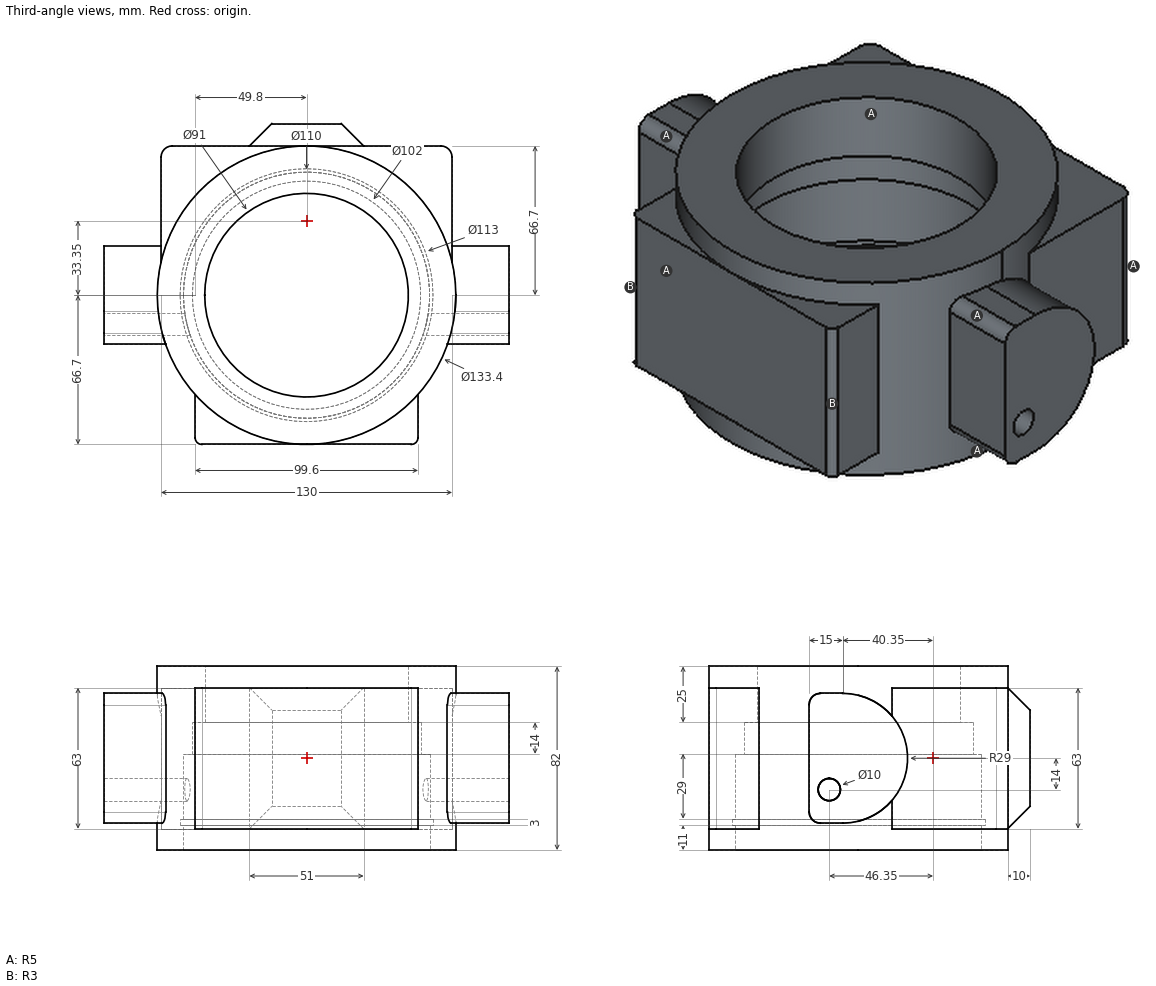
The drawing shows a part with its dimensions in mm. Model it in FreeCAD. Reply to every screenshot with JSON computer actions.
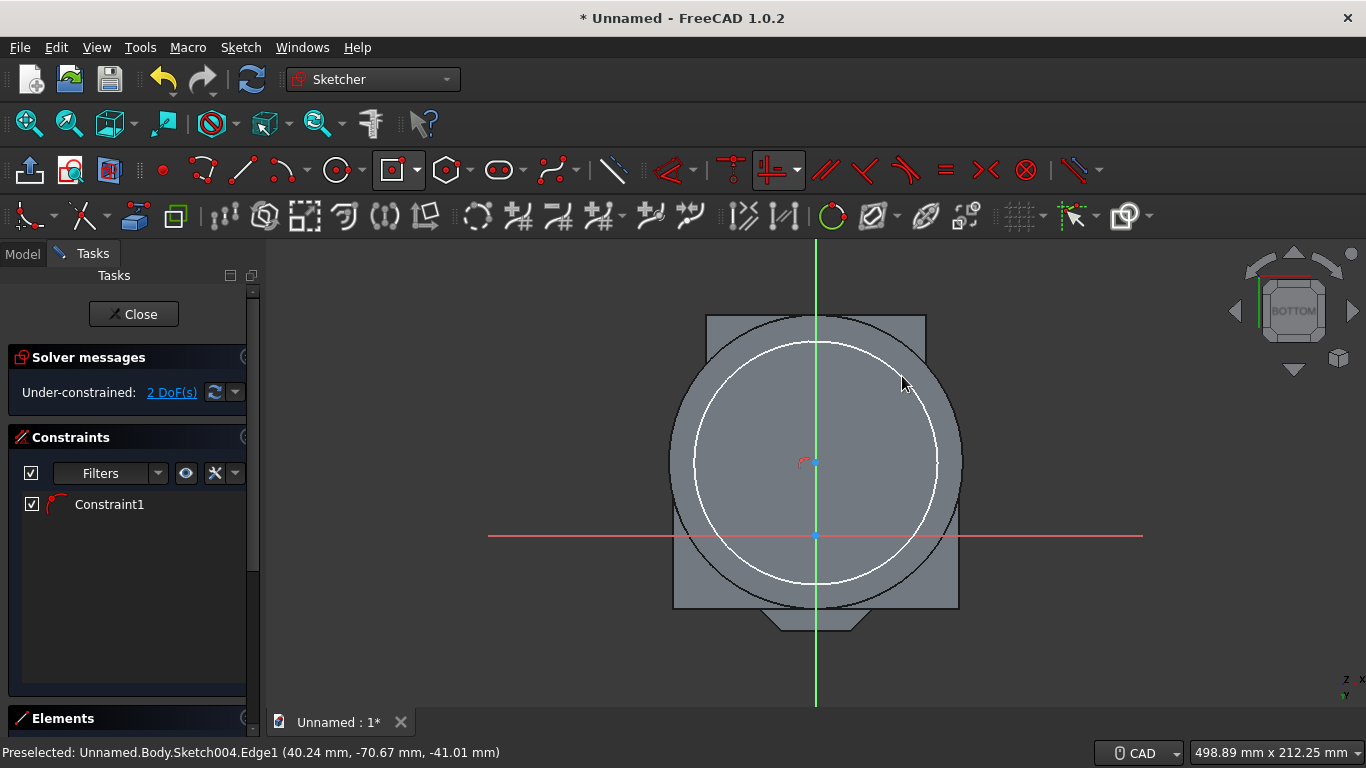
{"action": "key", "text": "d"}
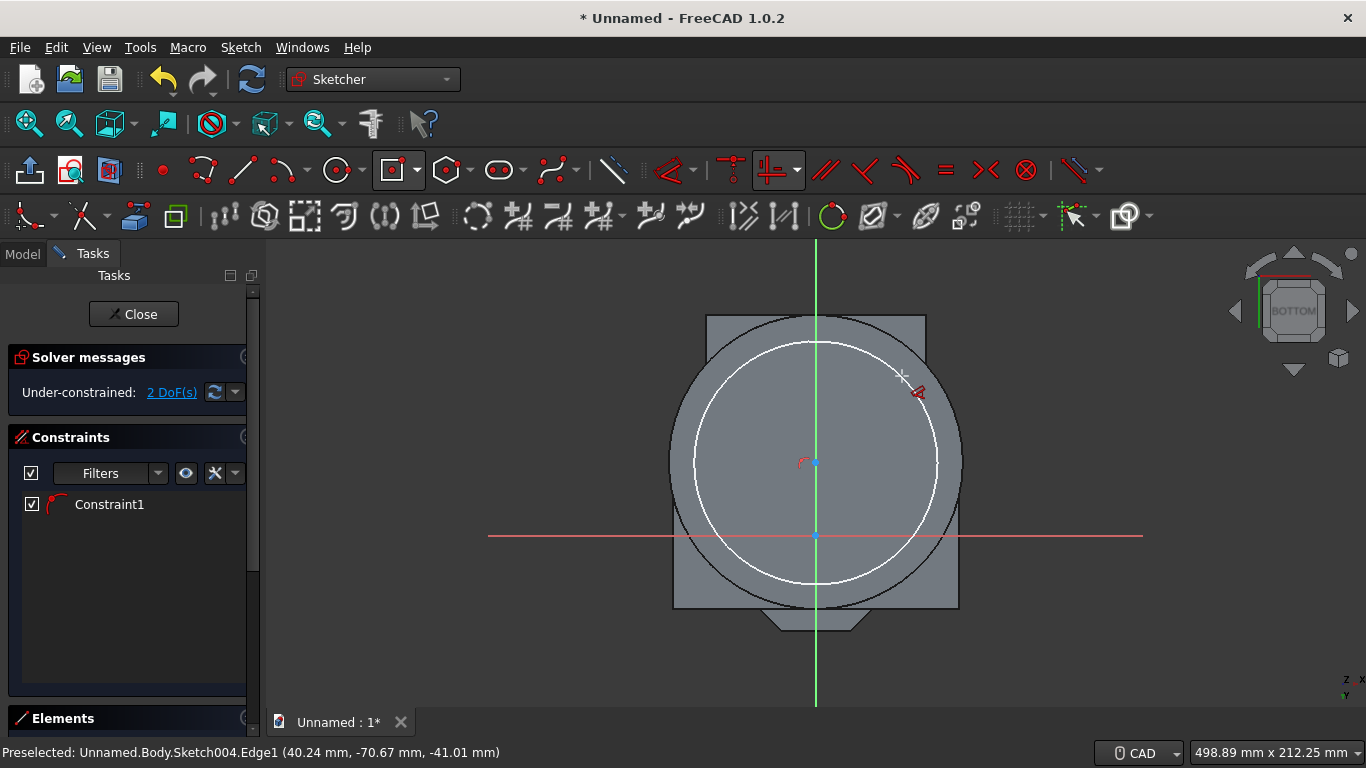
{"action": "left_click", "coordinate": [902, 377]}
{"action": "left_click", "coordinate": [925, 354]}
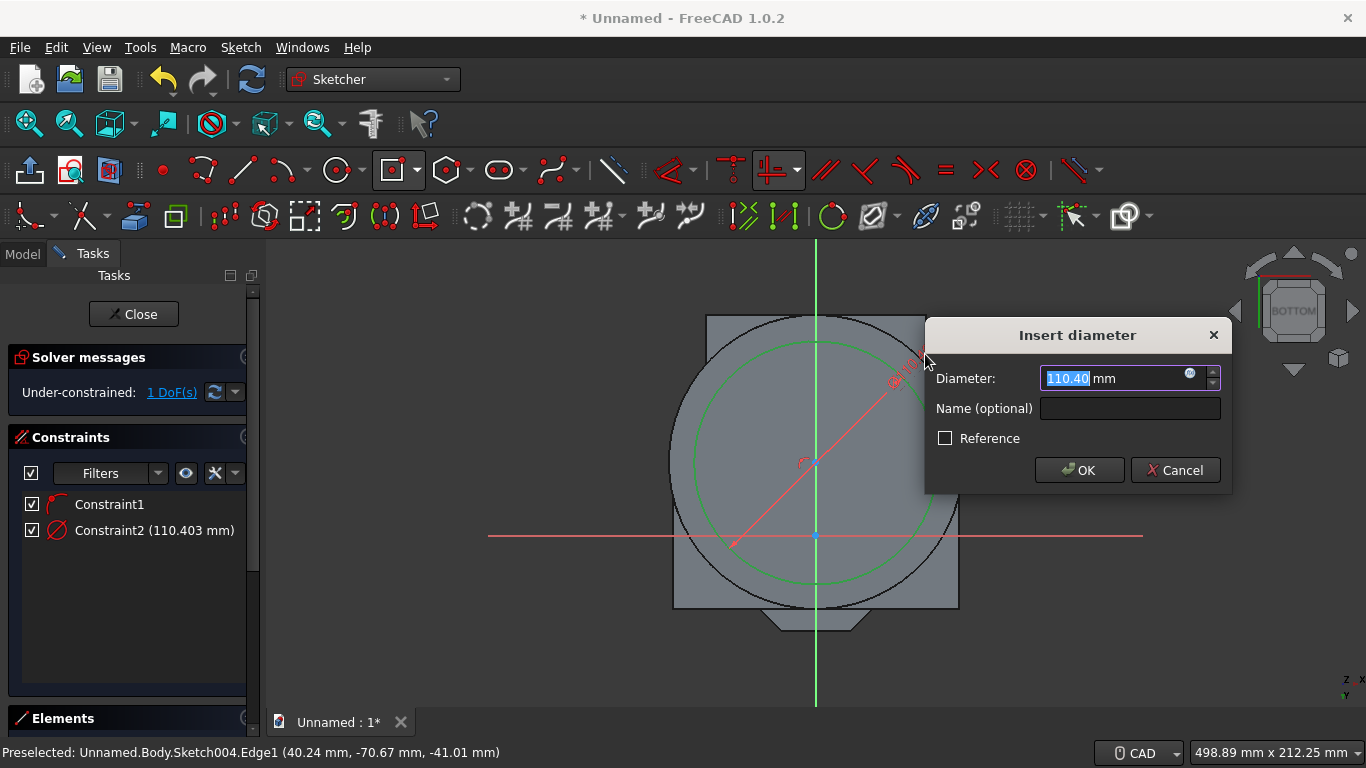
{"action": "type", "text": "110"}
{"action": "key", "text": "Return"}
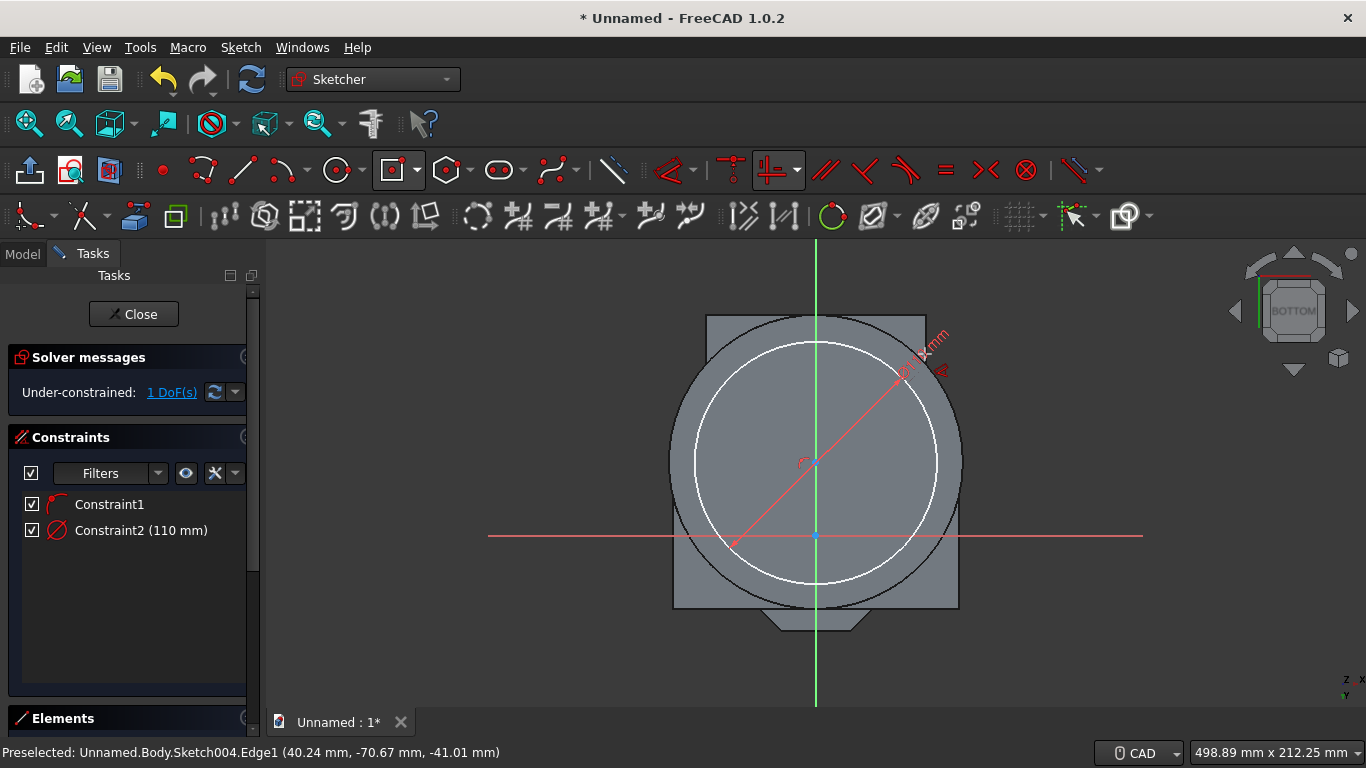
{"action": "left_click", "coordinate": [816, 463]}
{"action": "left_click", "coordinate": [850, 499]}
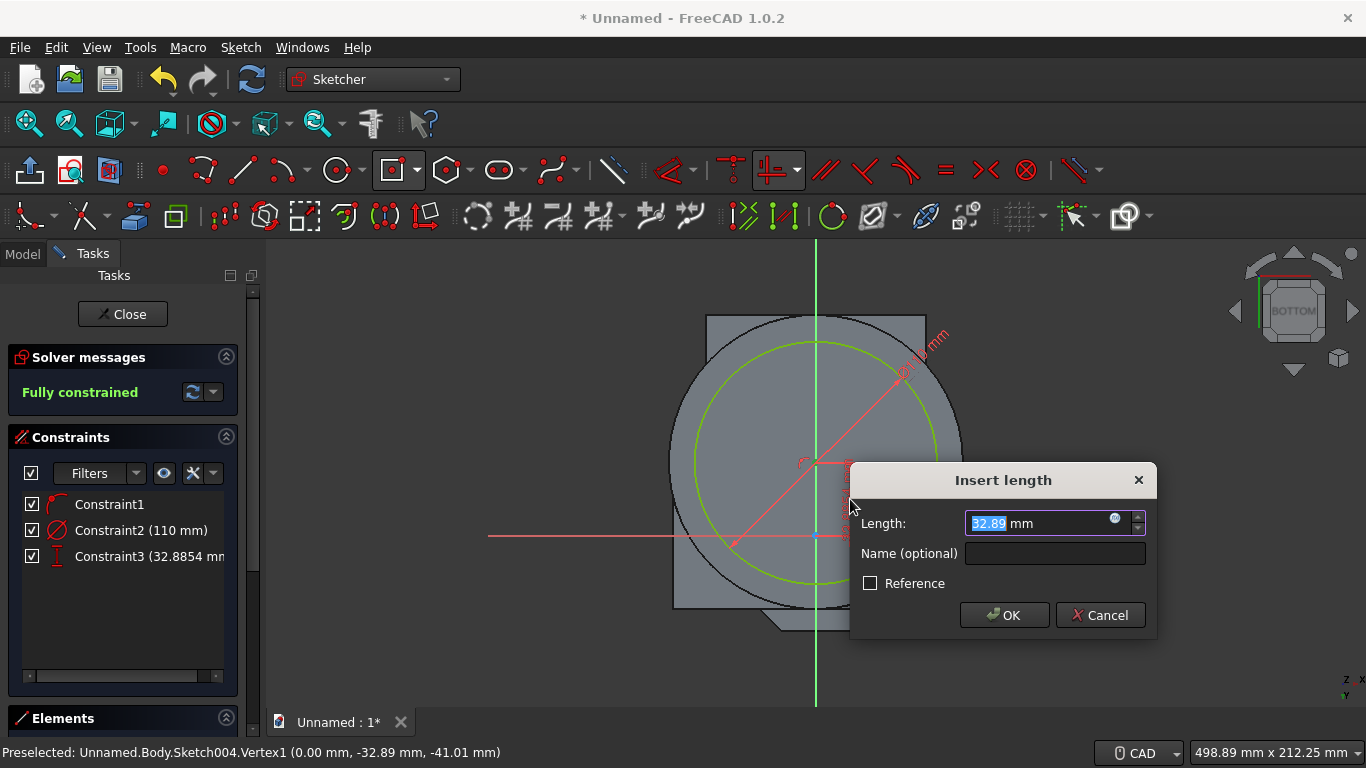
{"action": "type", "text": "33.35"}
{"action": "key", "text": "Return"}
{"action": "key", "text": "Escape"}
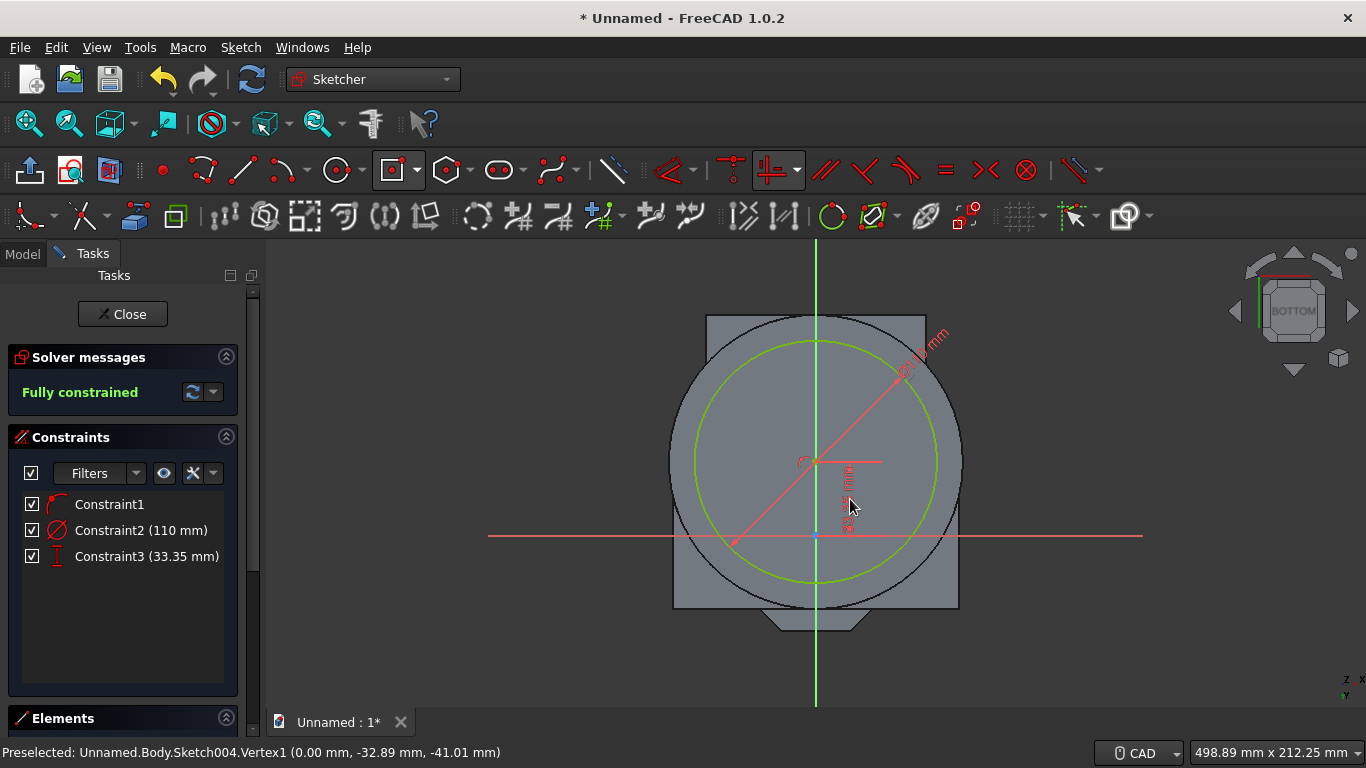
{"action": "left_click", "coordinate": [123, 314]}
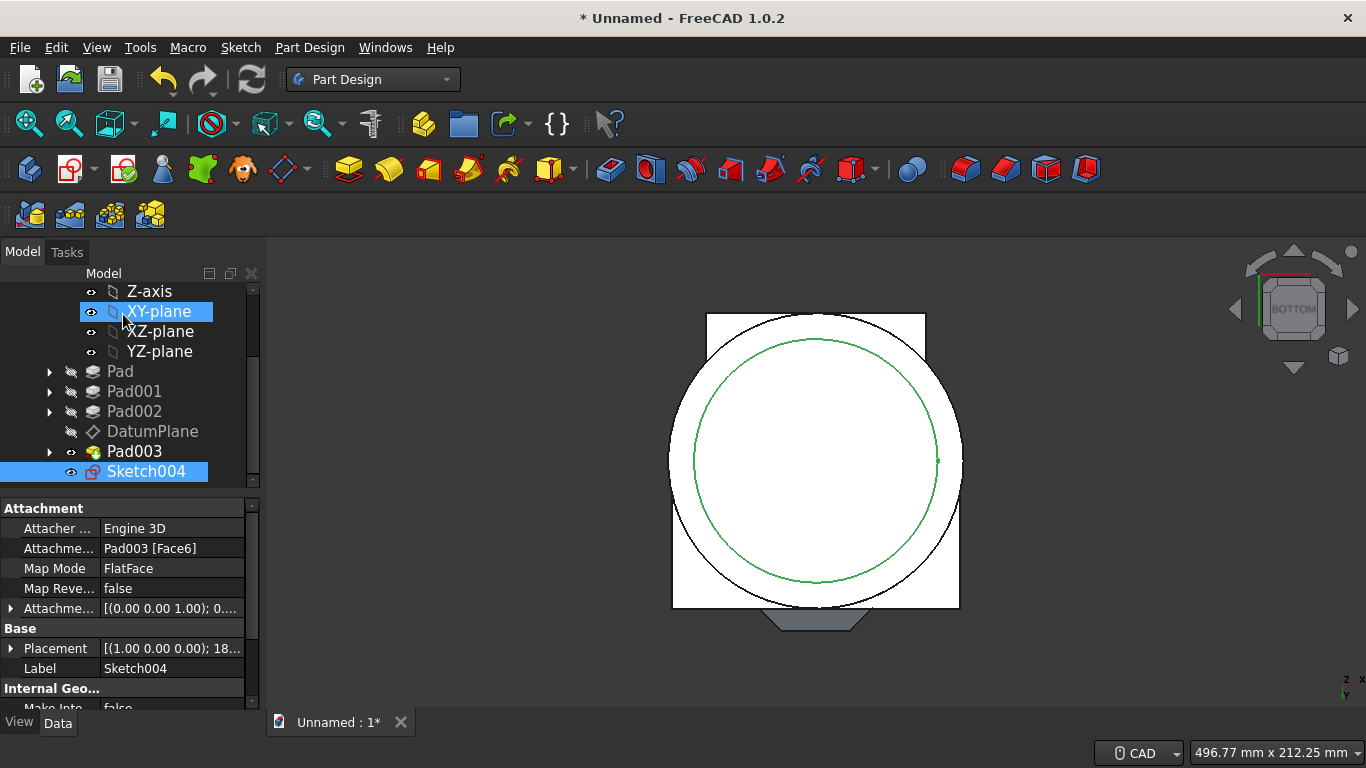
{"action": "left_click", "coordinate": [612, 170]}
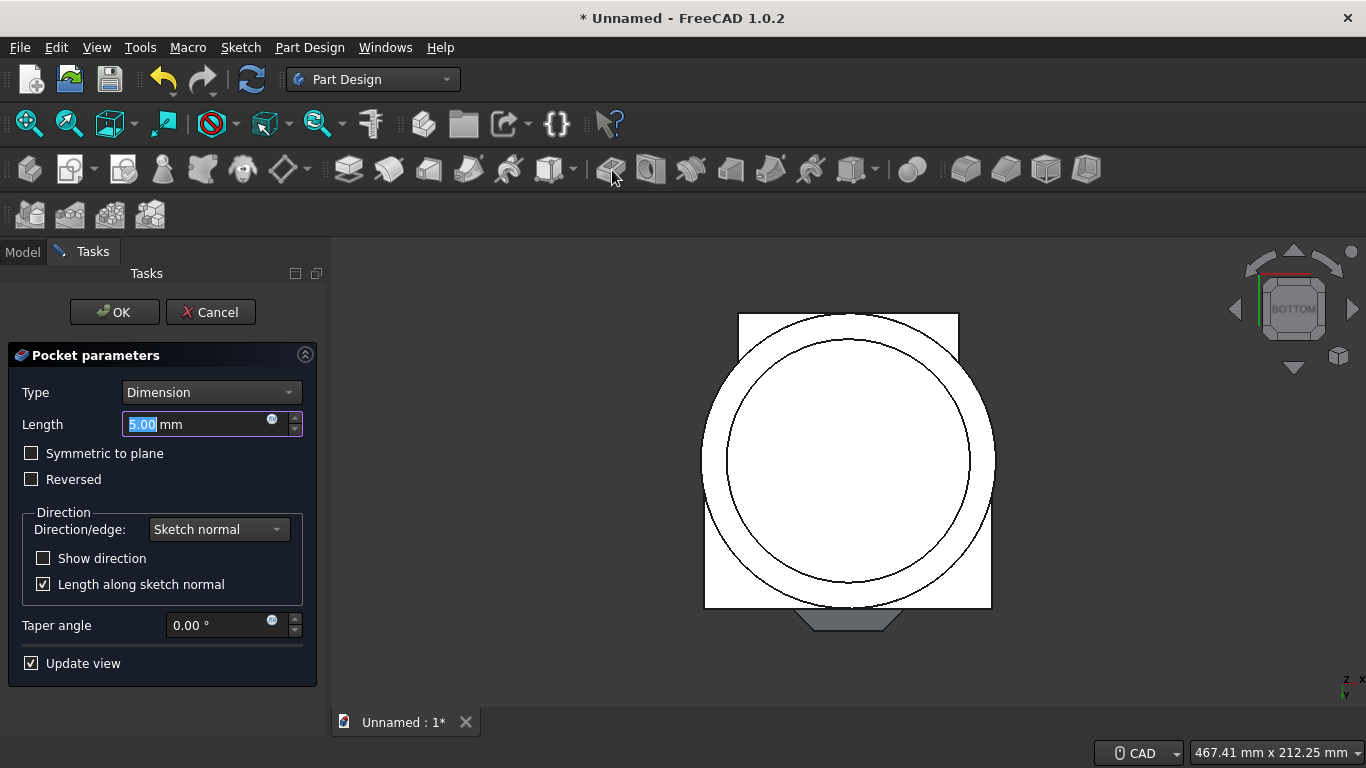
{"action": "type", "text": "11"}
{"action": "key", "text": "Tab"}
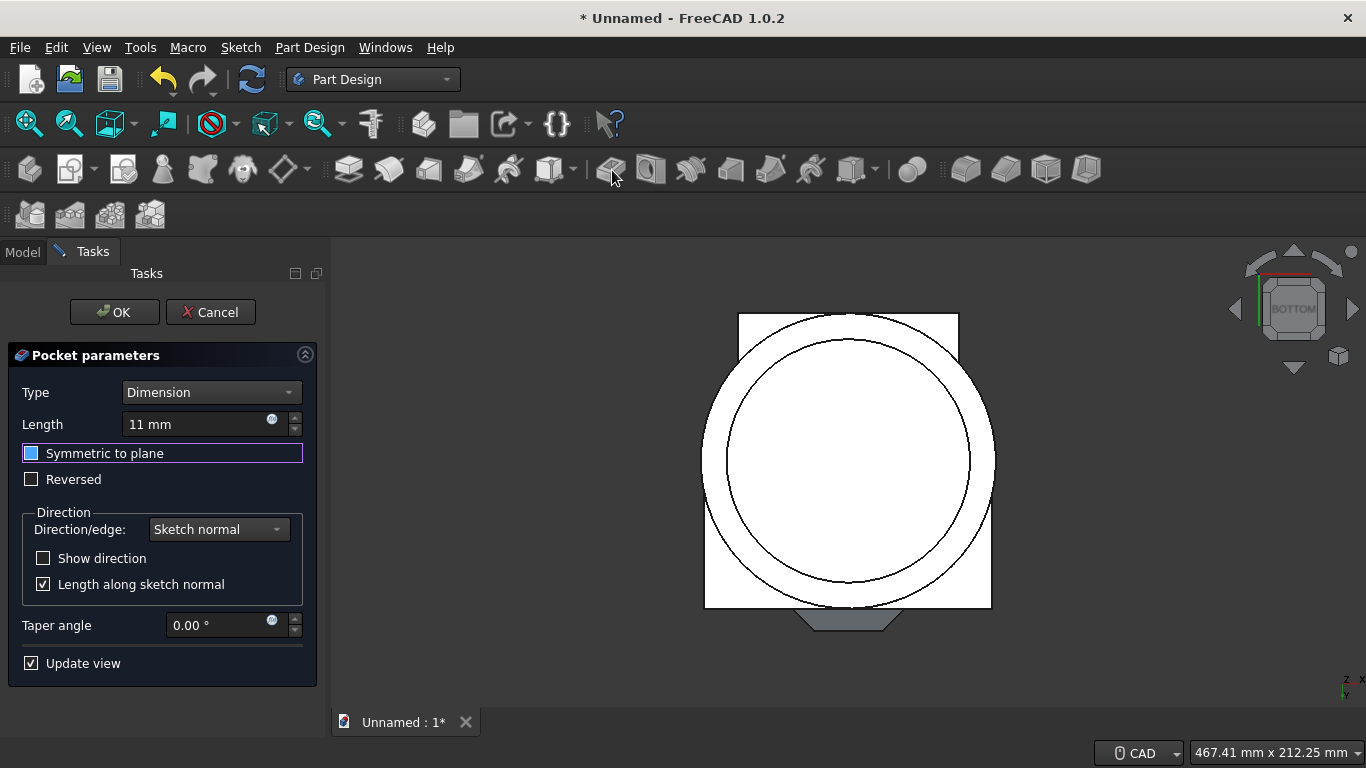
{"action": "left_click", "coordinate": [115, 312]}